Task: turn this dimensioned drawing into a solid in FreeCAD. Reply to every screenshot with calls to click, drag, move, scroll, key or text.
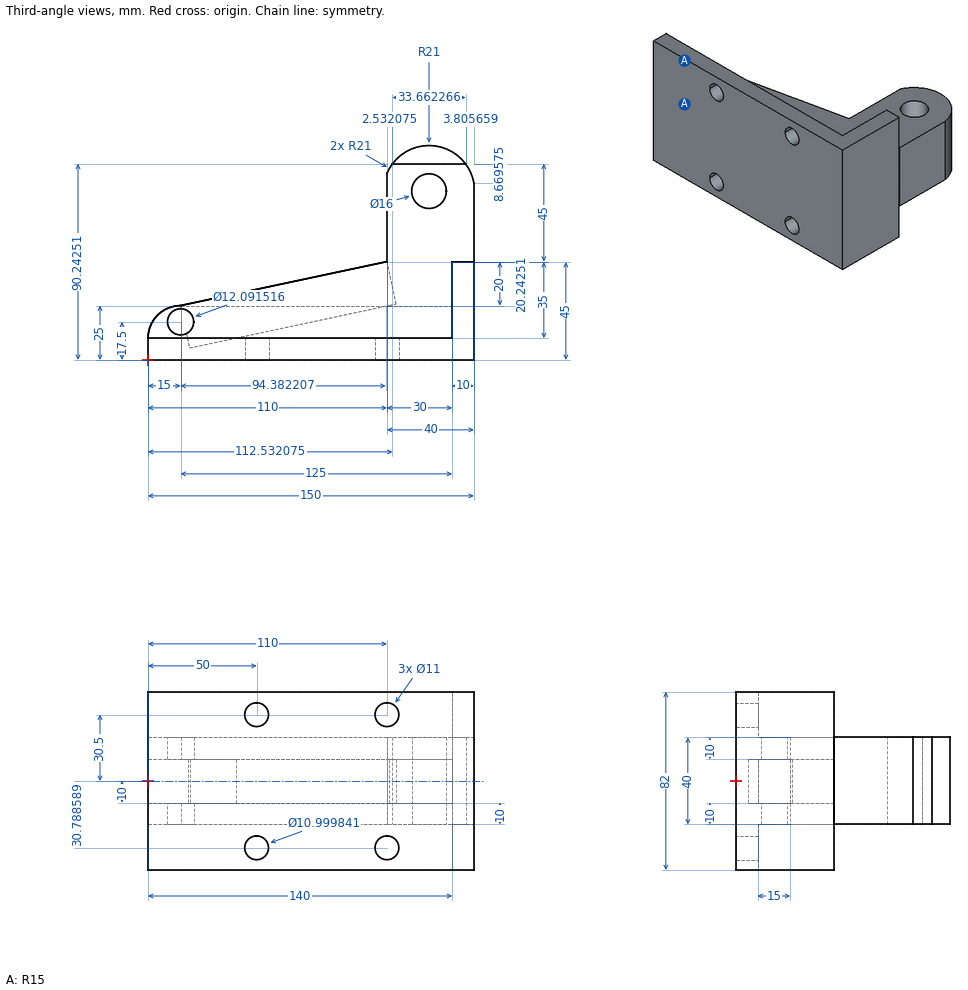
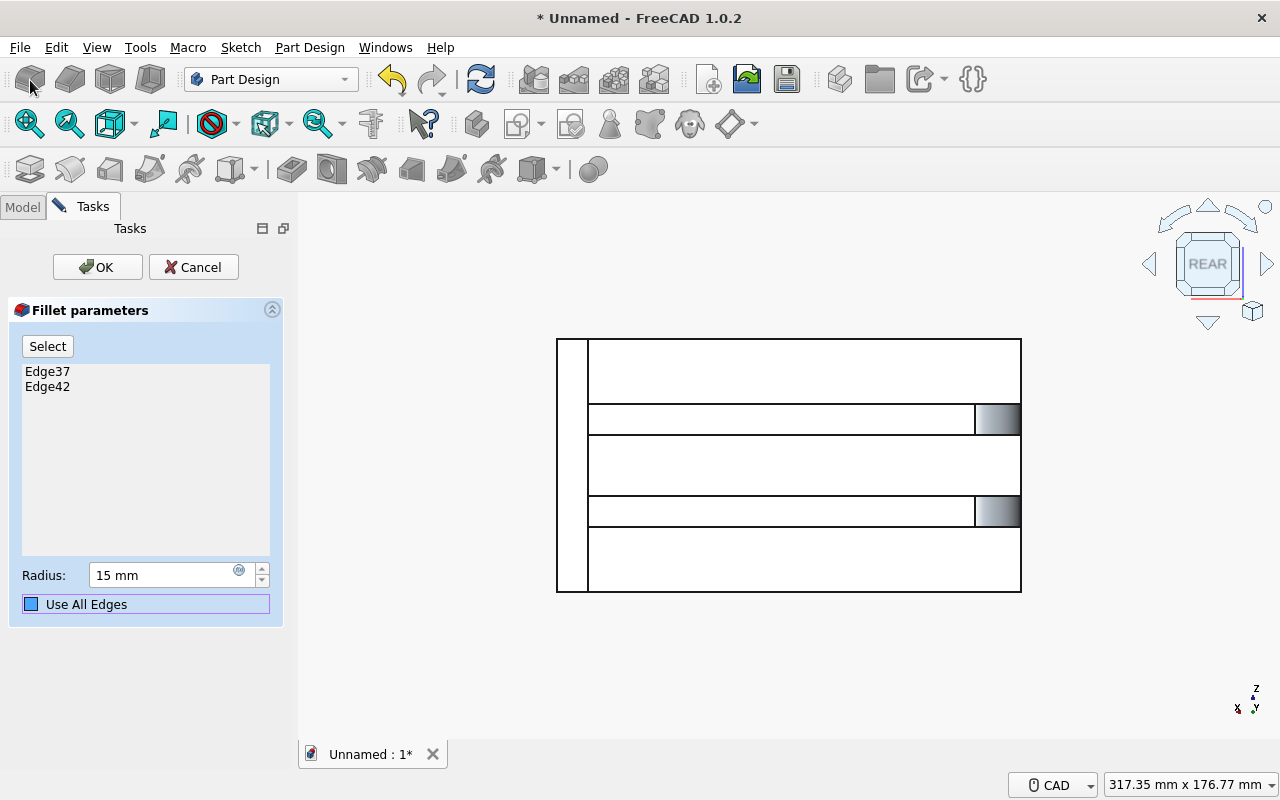
click(98, 267)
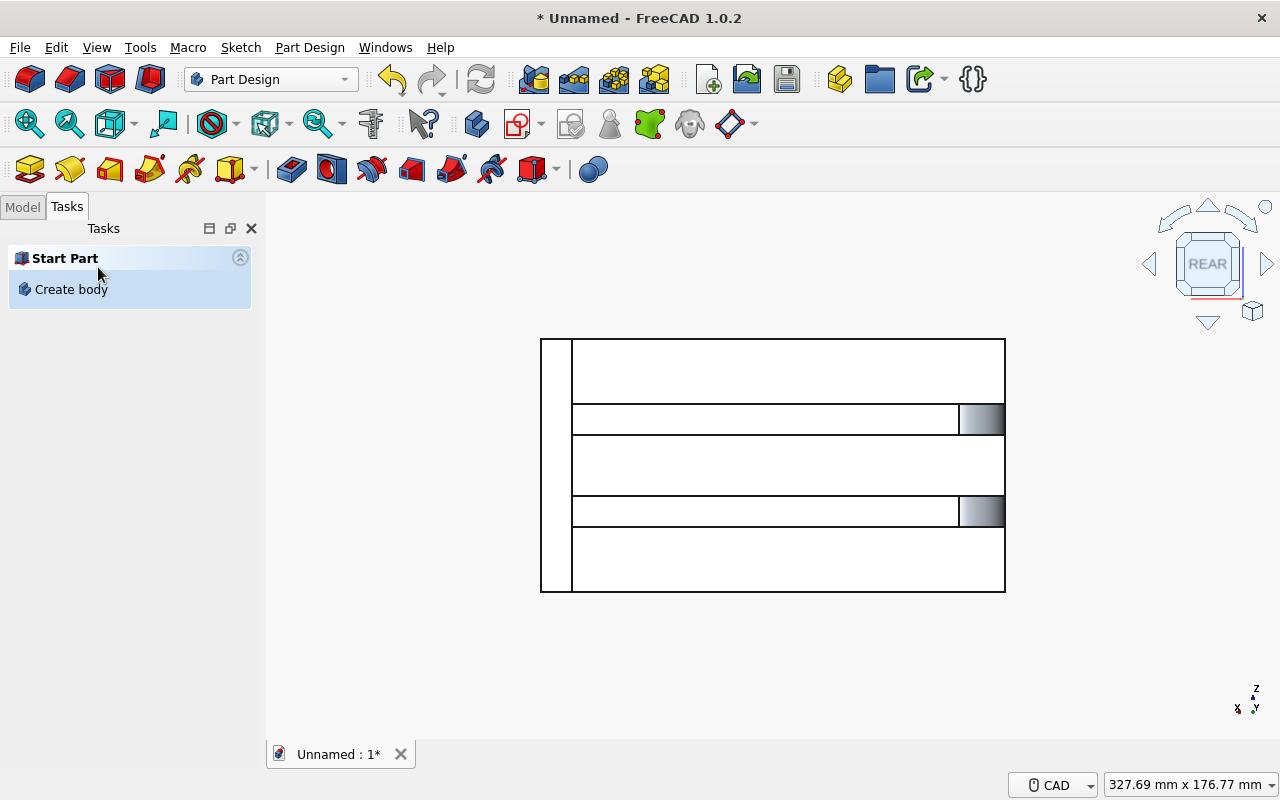
key(0)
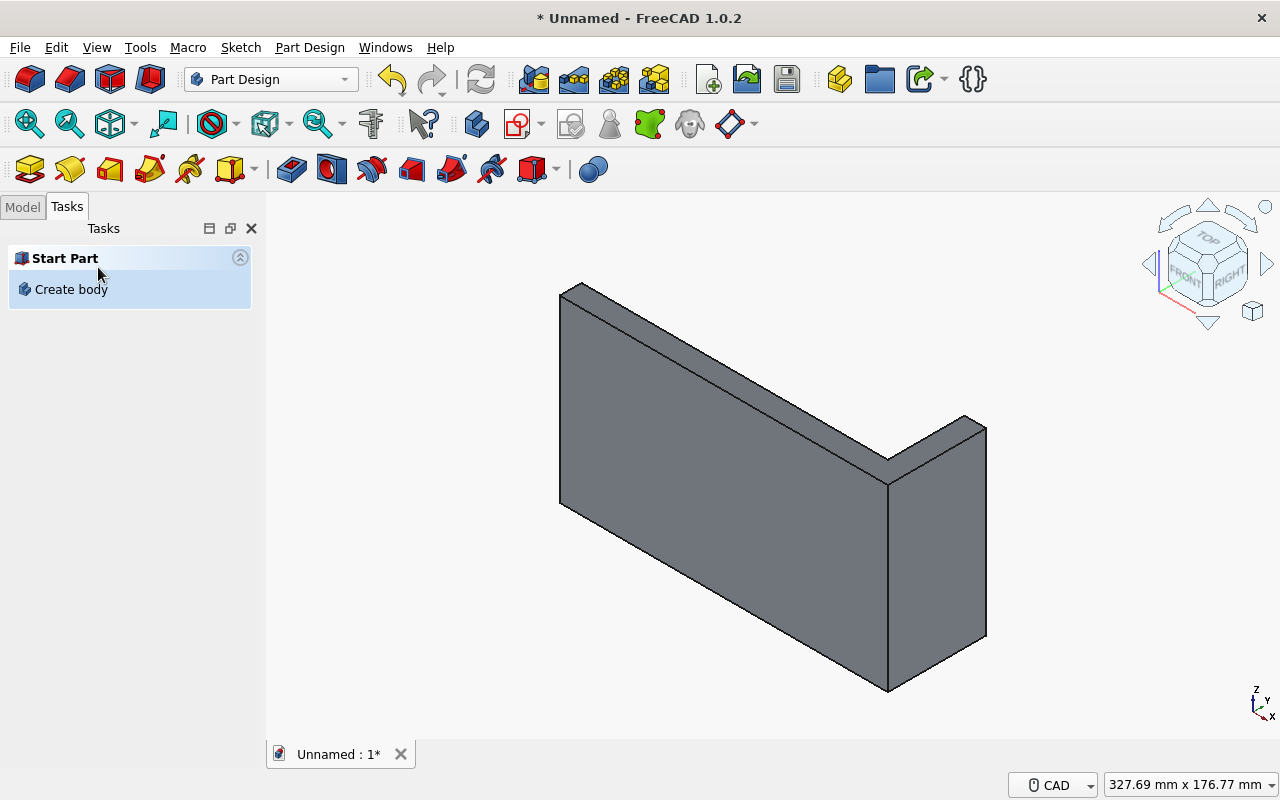
key(2)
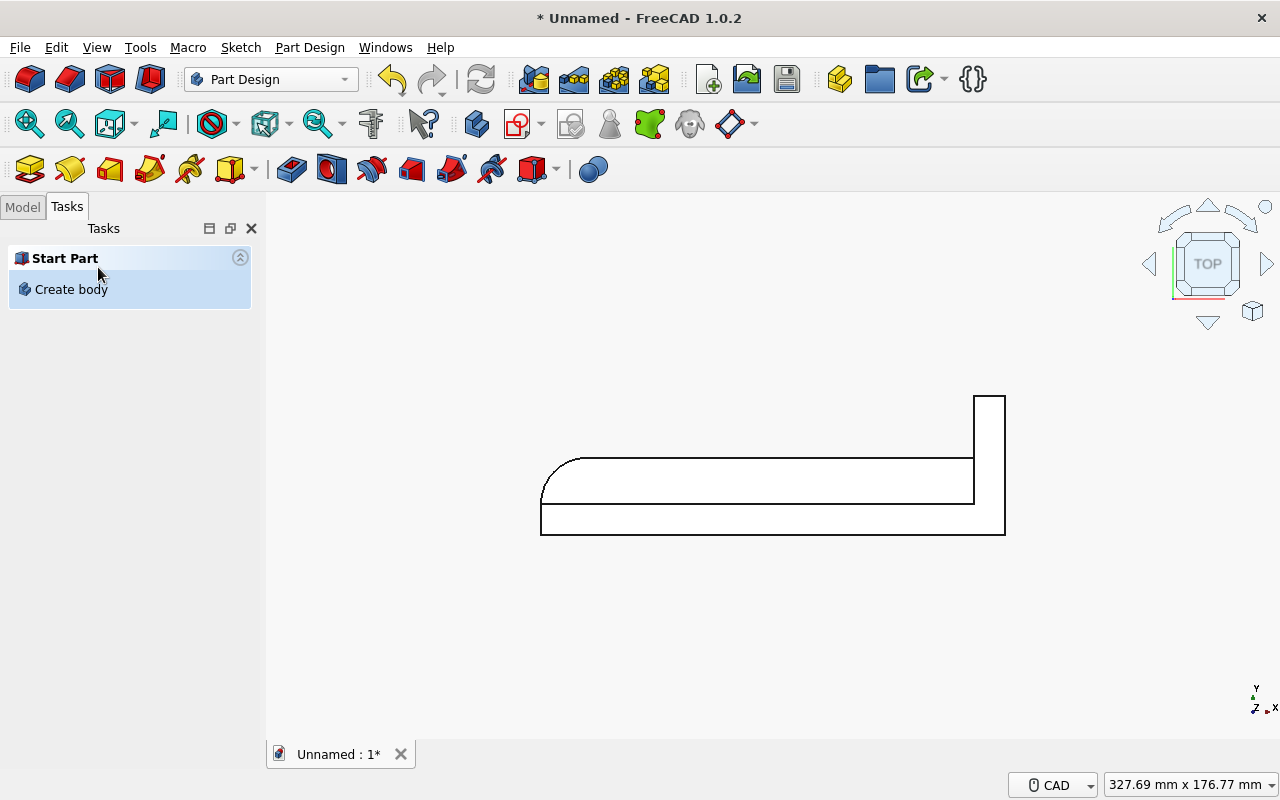
click(943, 480)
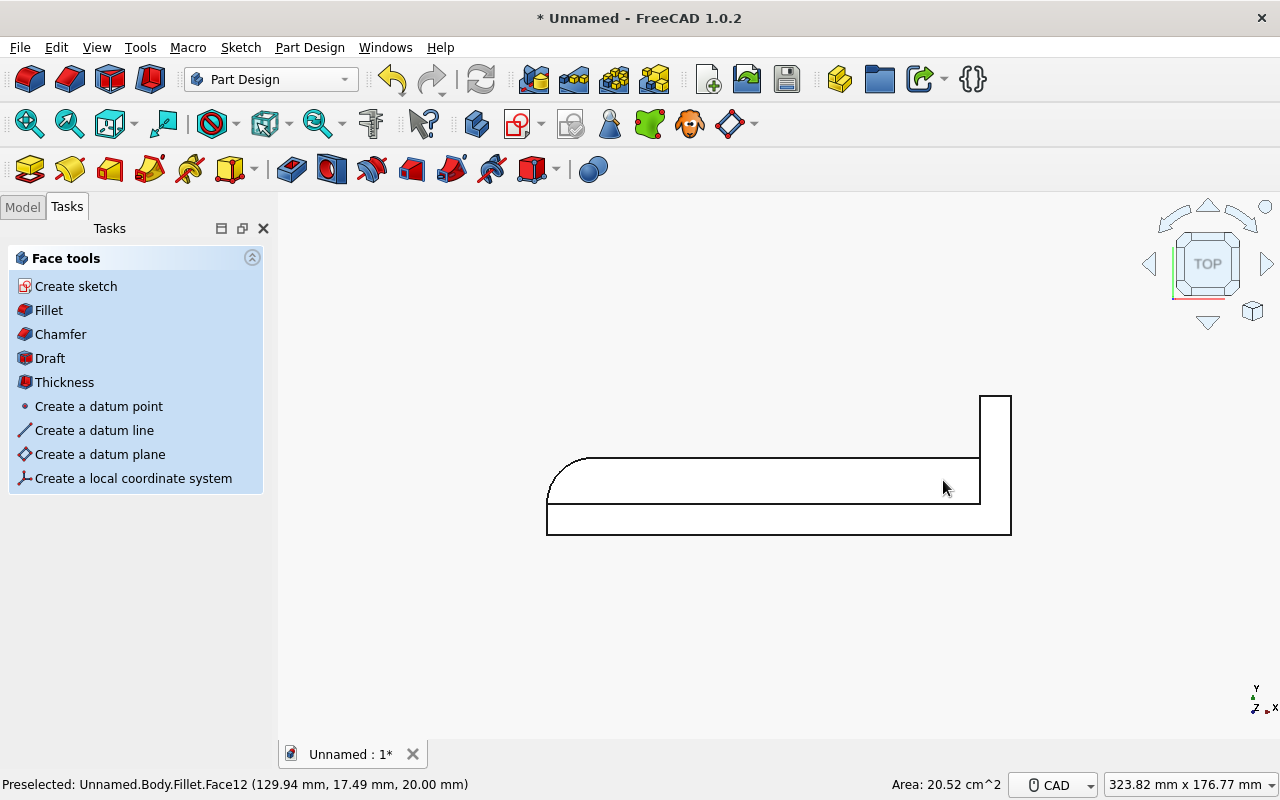
click(518, 124)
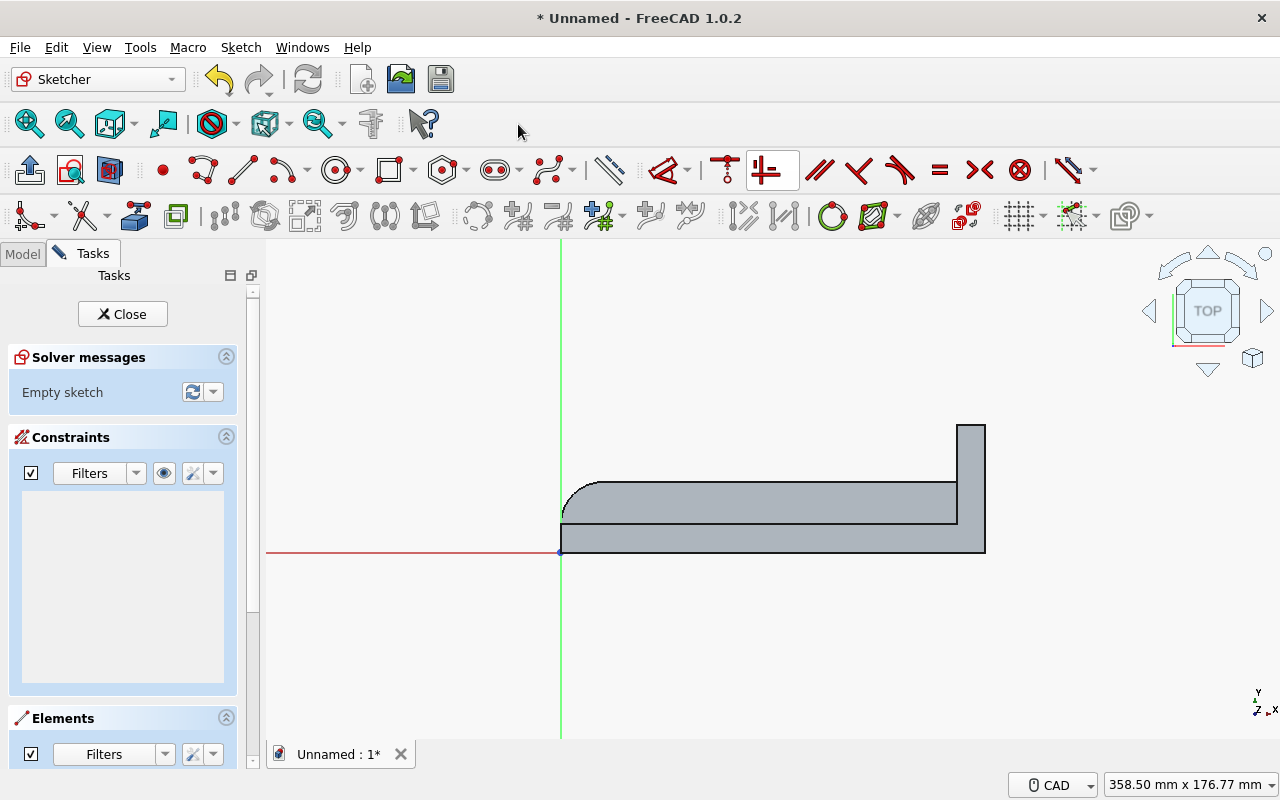
scroll(562, 527, up, 8)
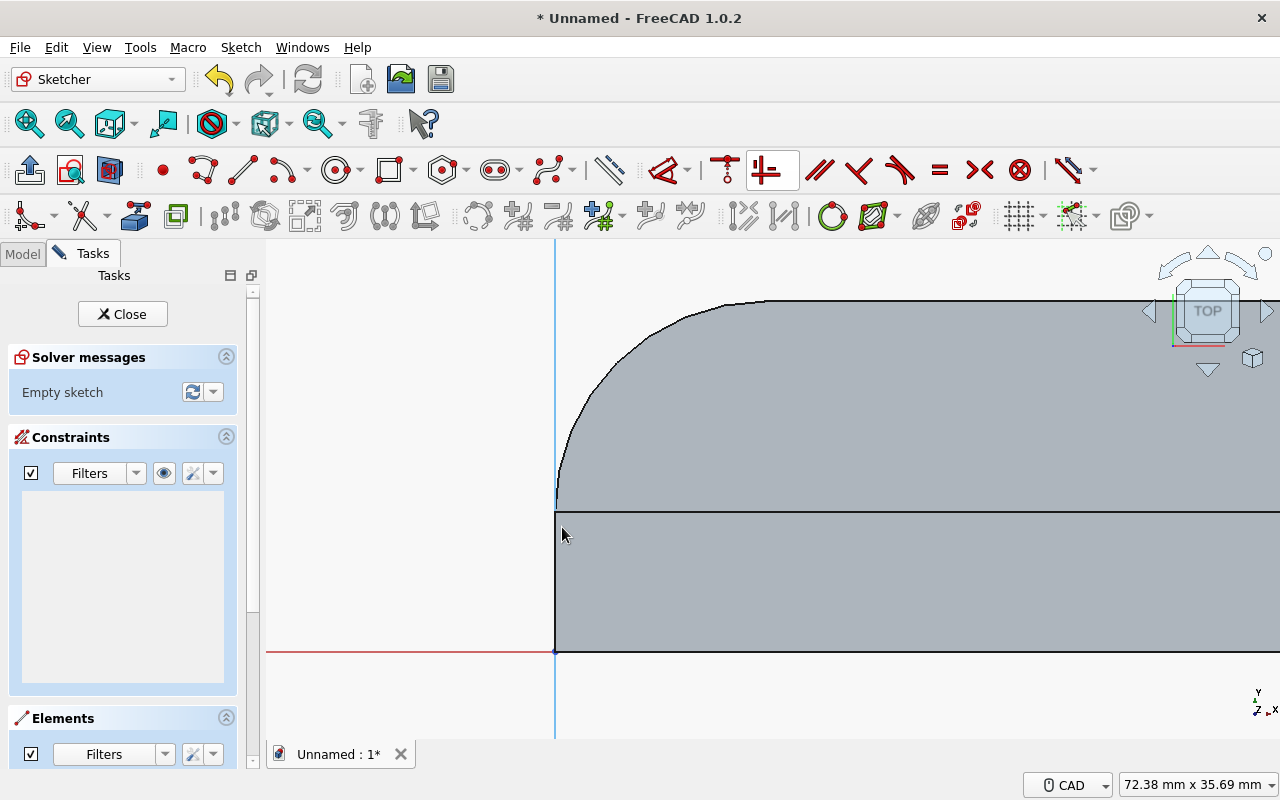
key(g)
key(c)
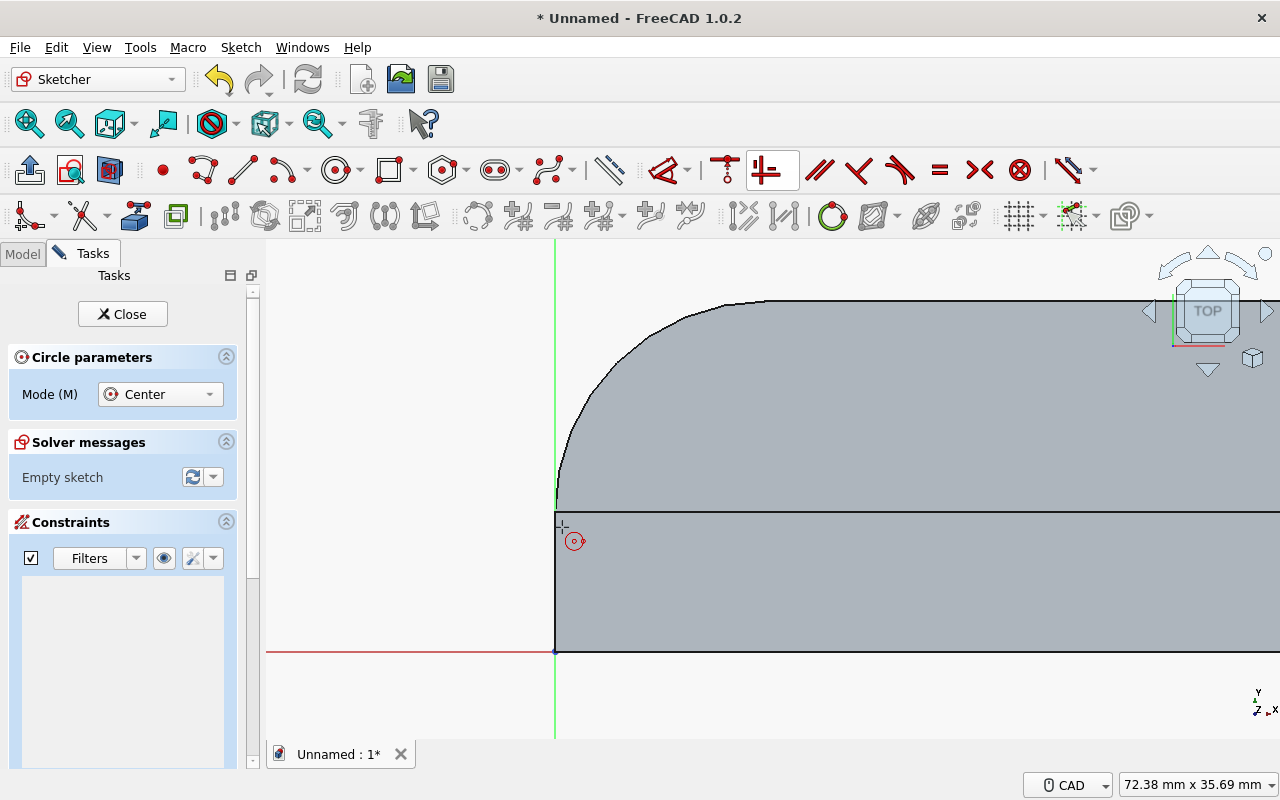
click(765, 407)
move(825, 347)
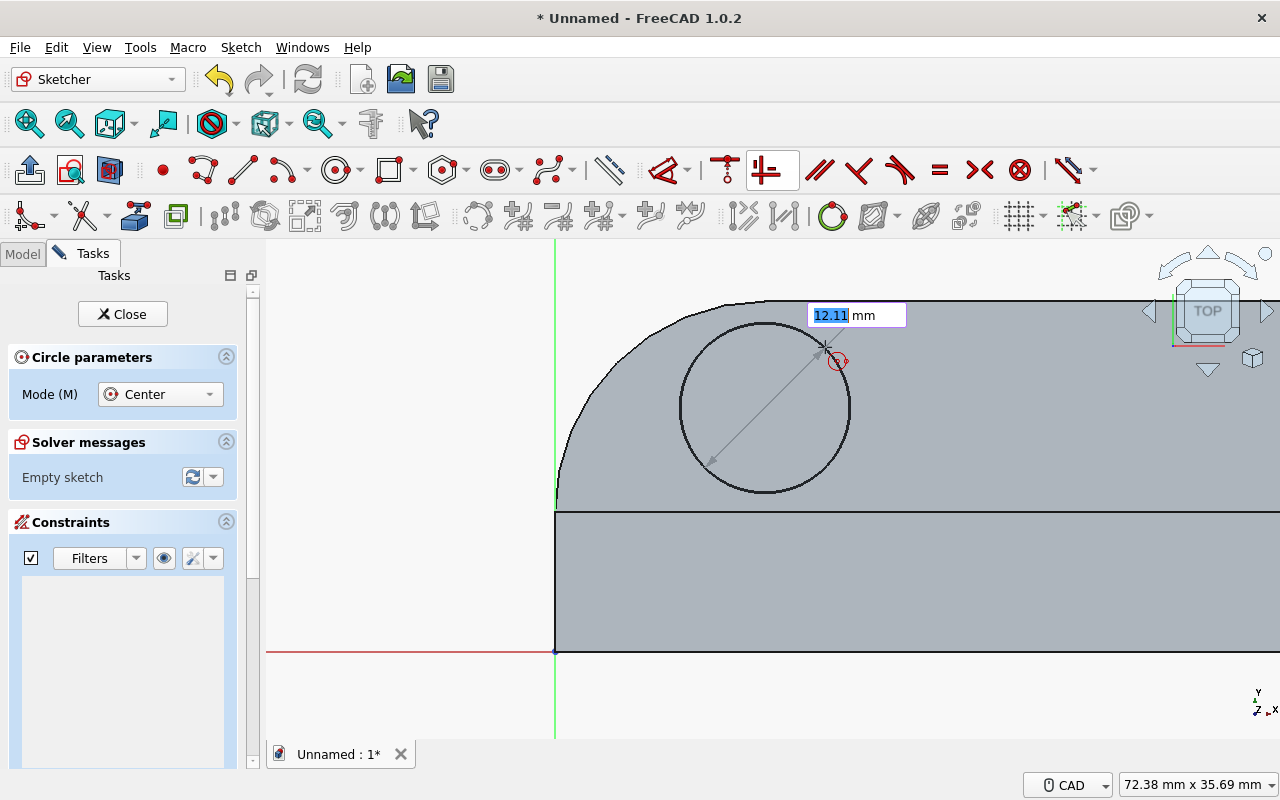
text(12.091516)
key(Return)
key(Escape)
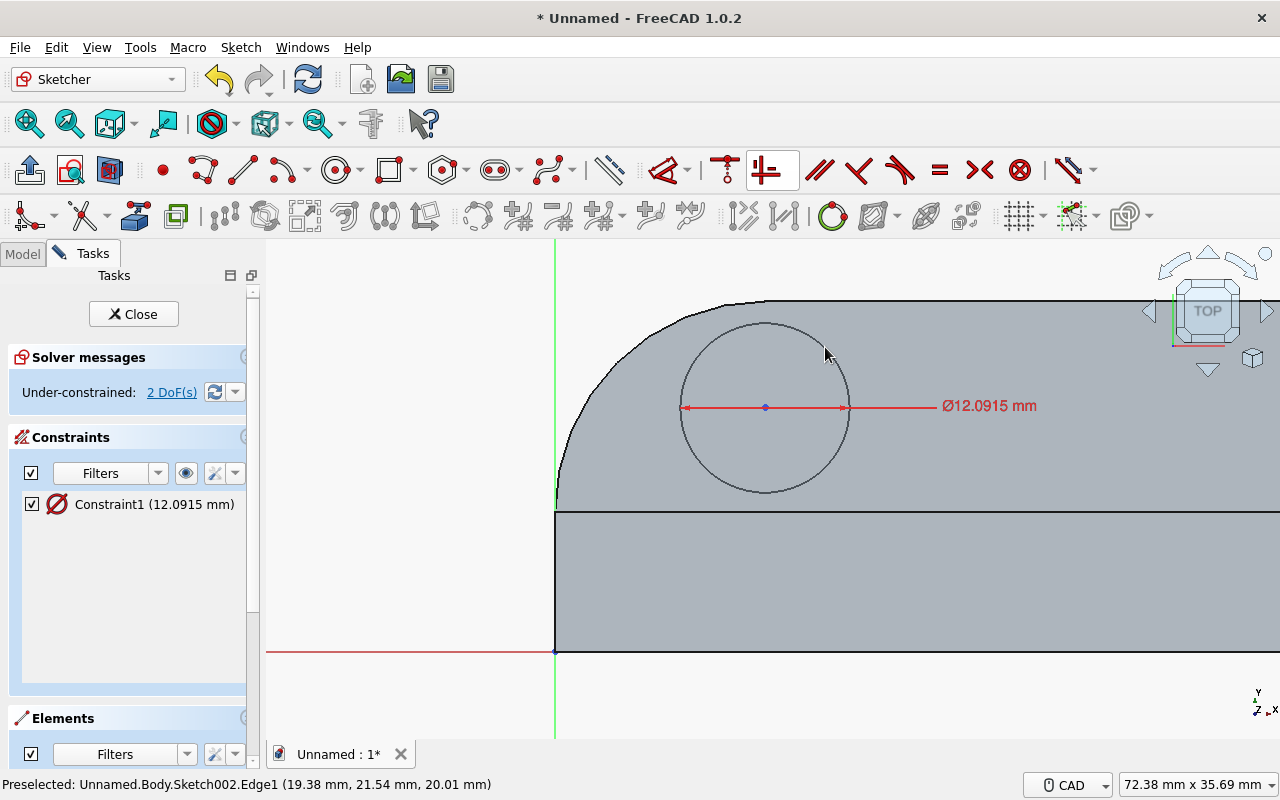
key(d)